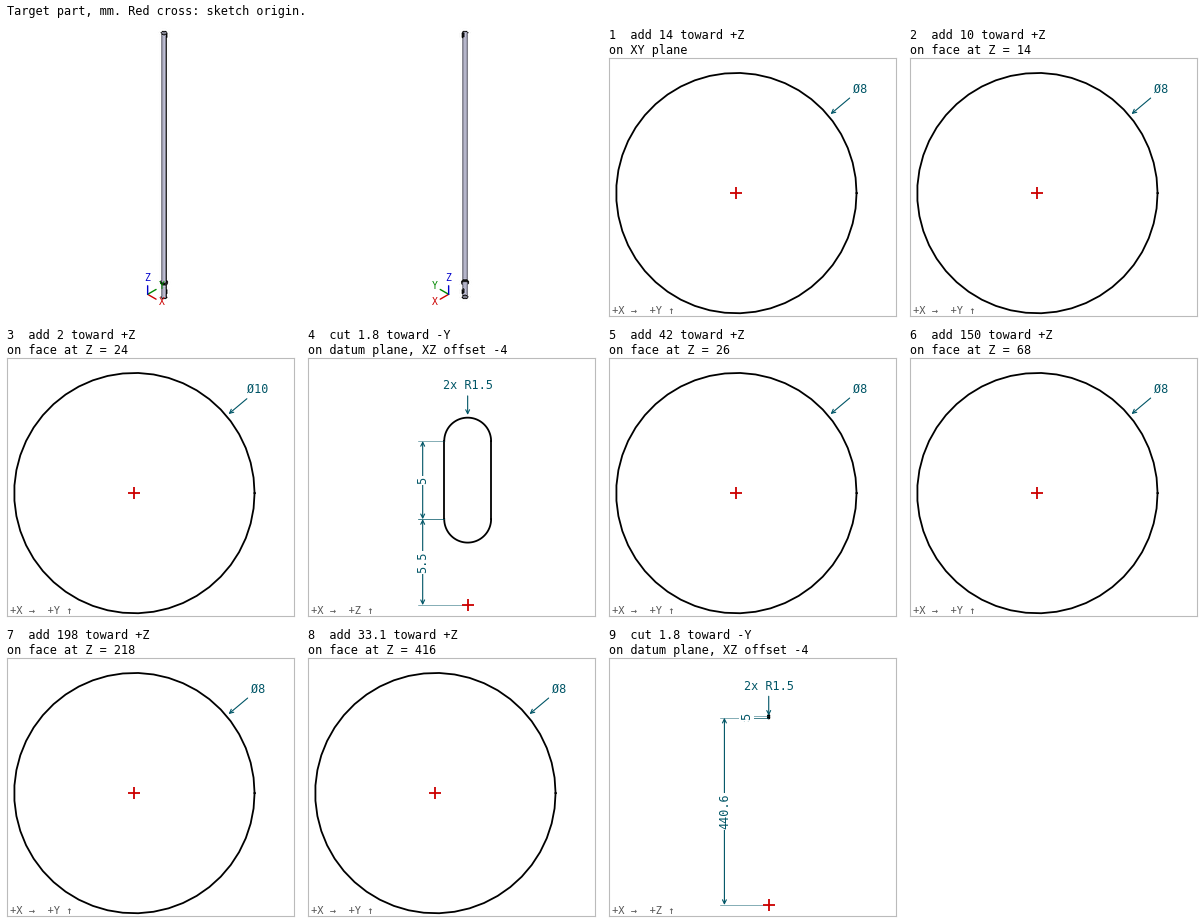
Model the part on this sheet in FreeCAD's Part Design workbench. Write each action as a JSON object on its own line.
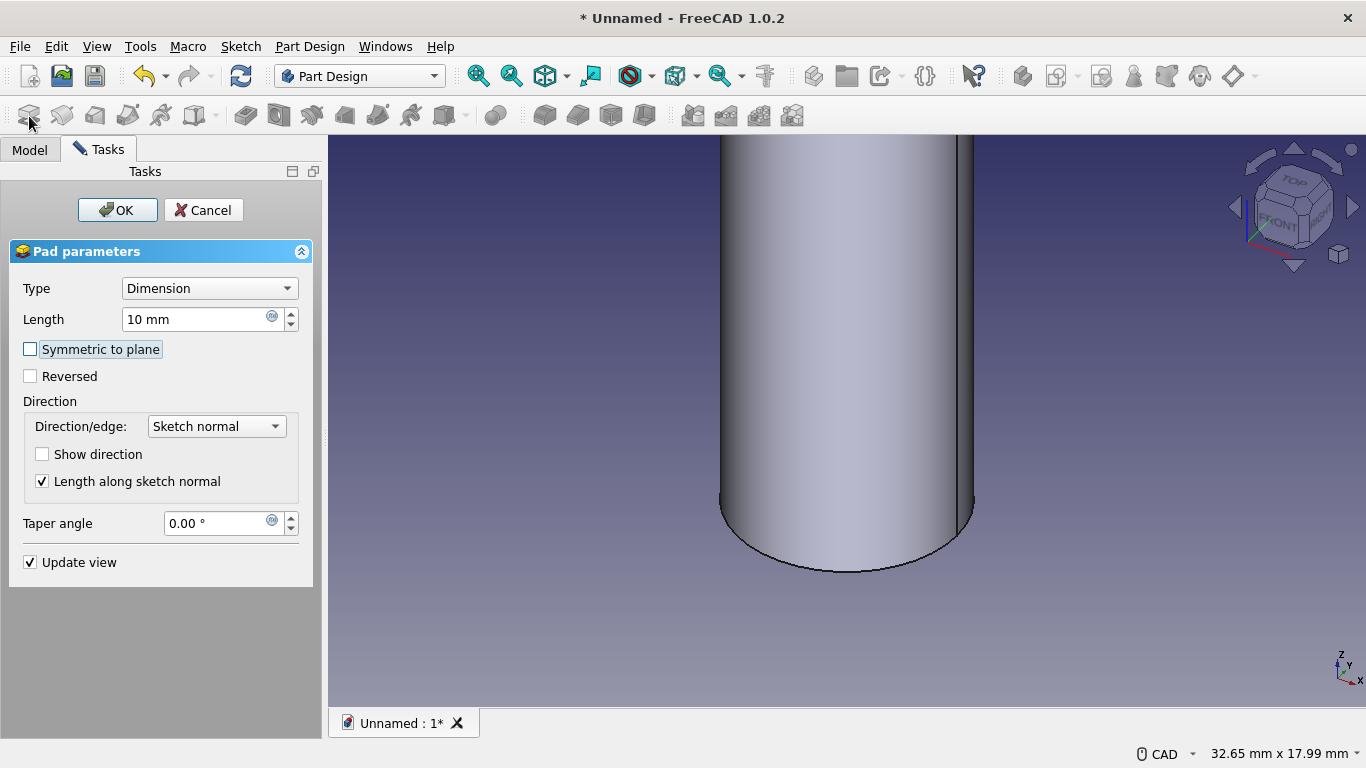
{"action": "left_click", "coordinate": [118, 210]}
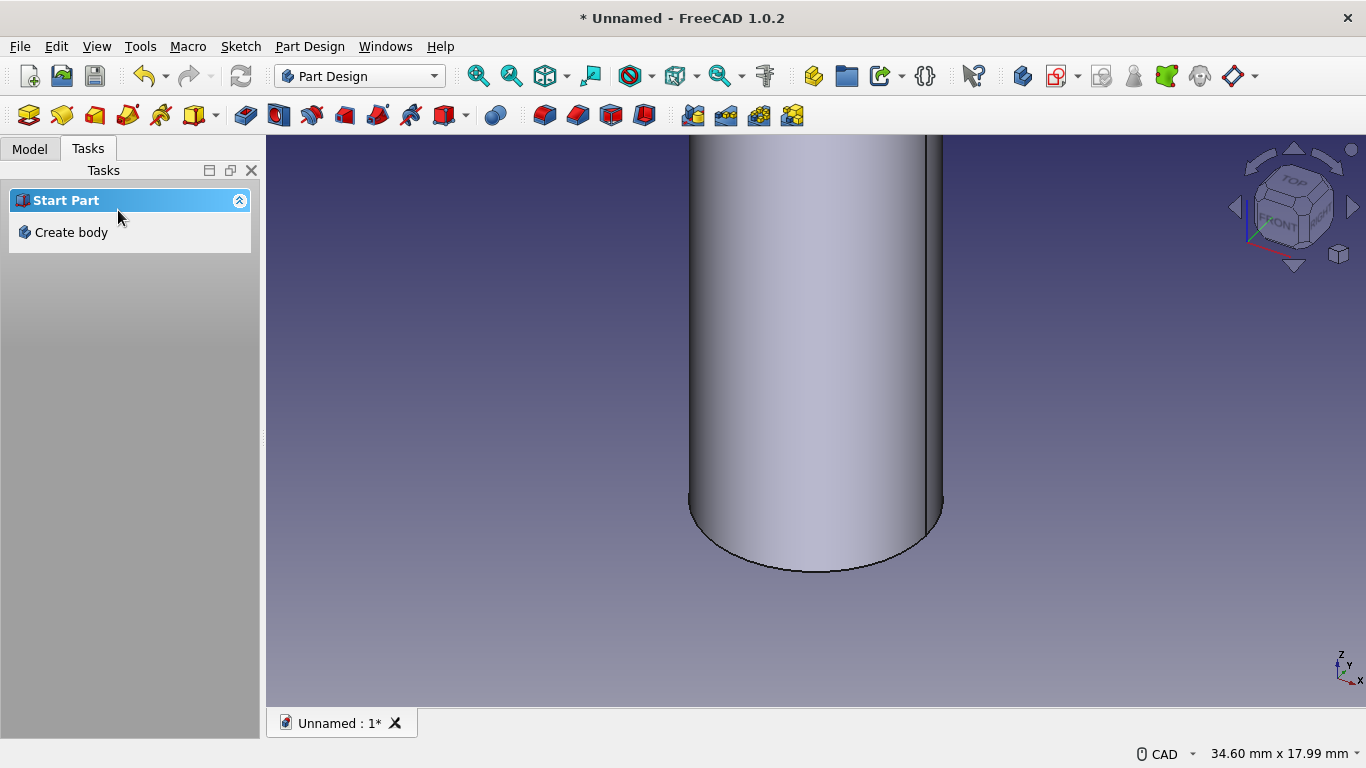
{"action": "left_click", "coordinate": [479, 76]}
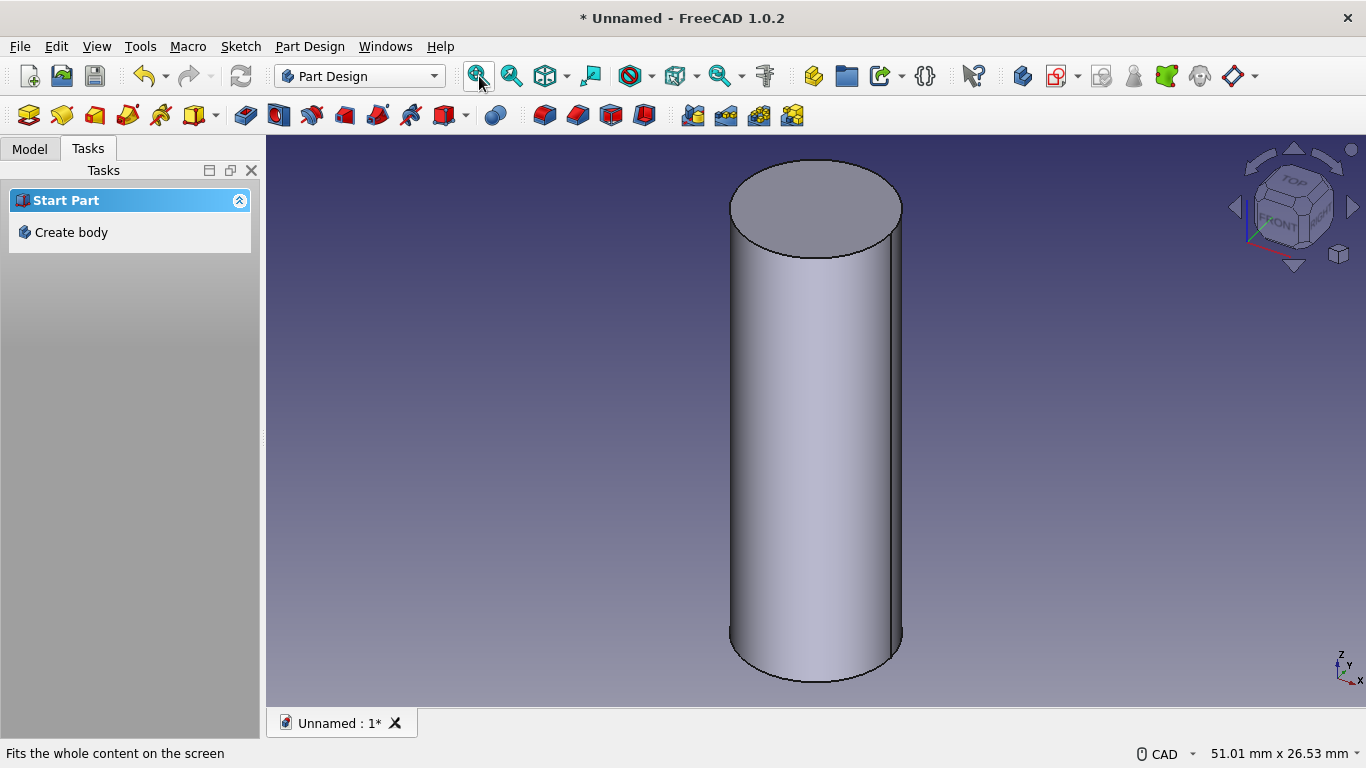
{"action": "left_click", "coordinate": [816, 208]}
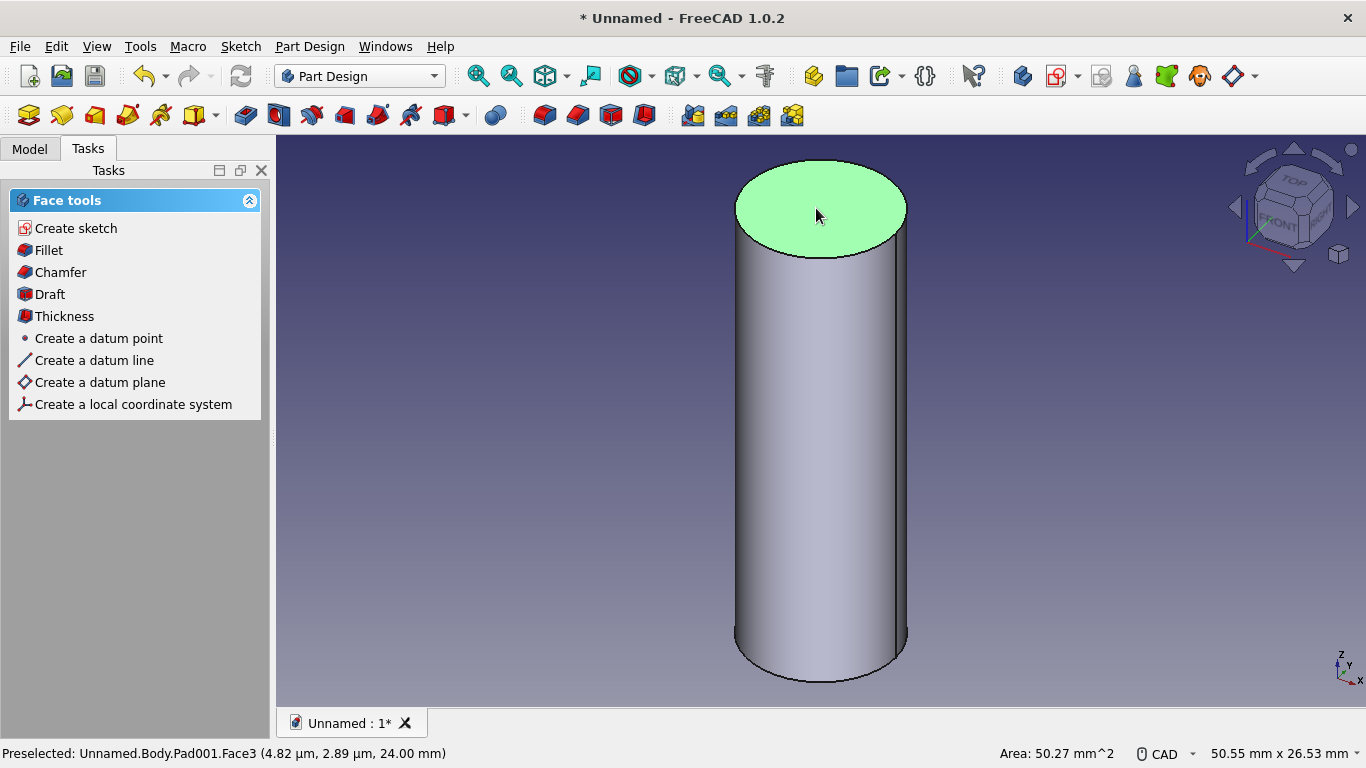
{"action": "left_click", "coordinate": [1056, 76]}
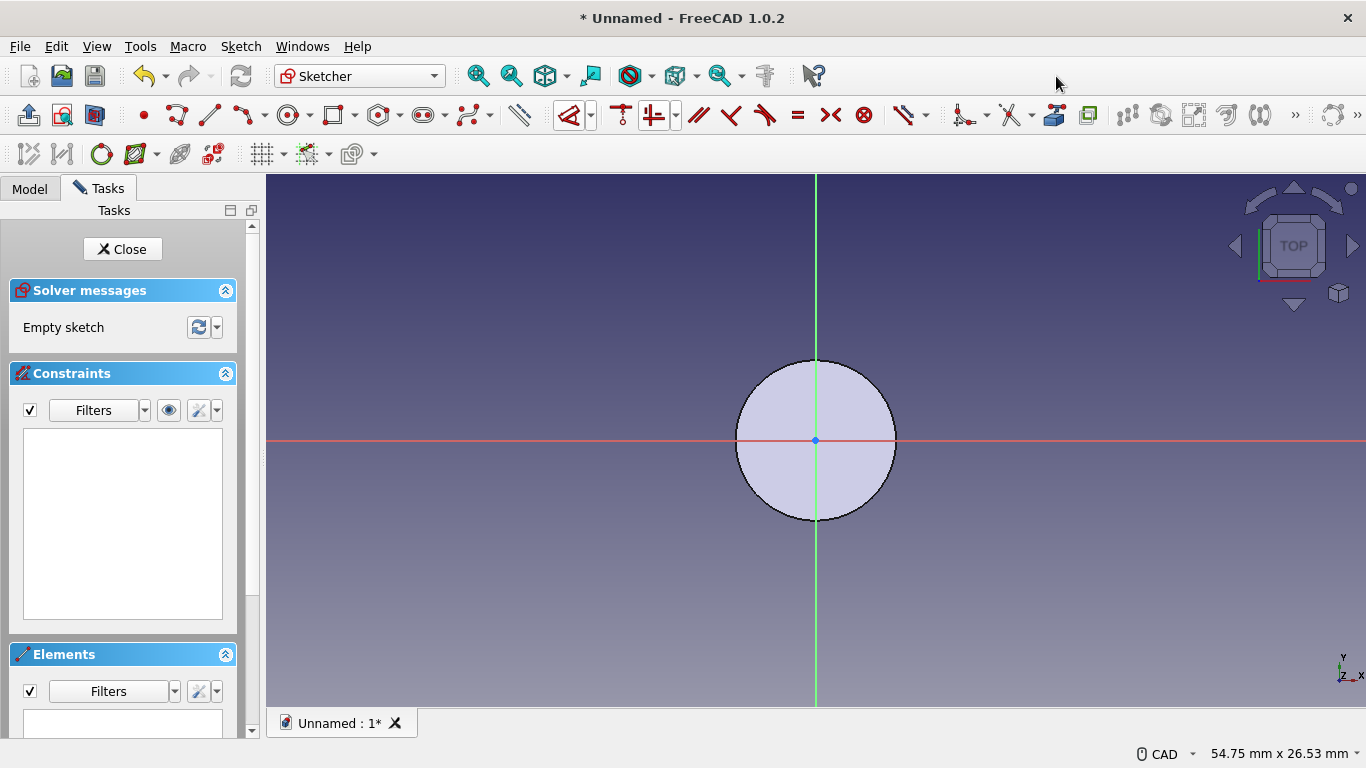
{"action": "scroll", "coordinate": [899, 441], "scroll_direction": "up", "scroll_amount": 3}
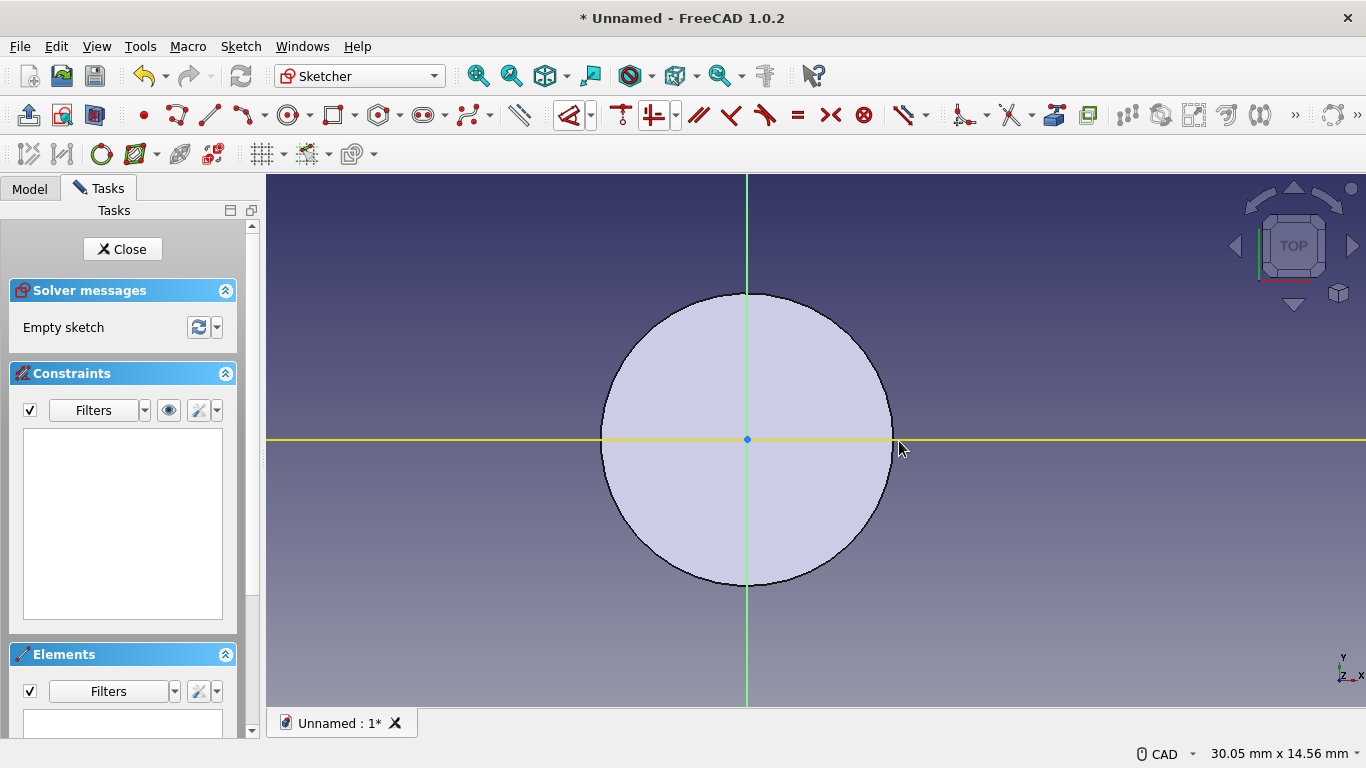
{"action": "left_click", "coordinate": [288, 116]}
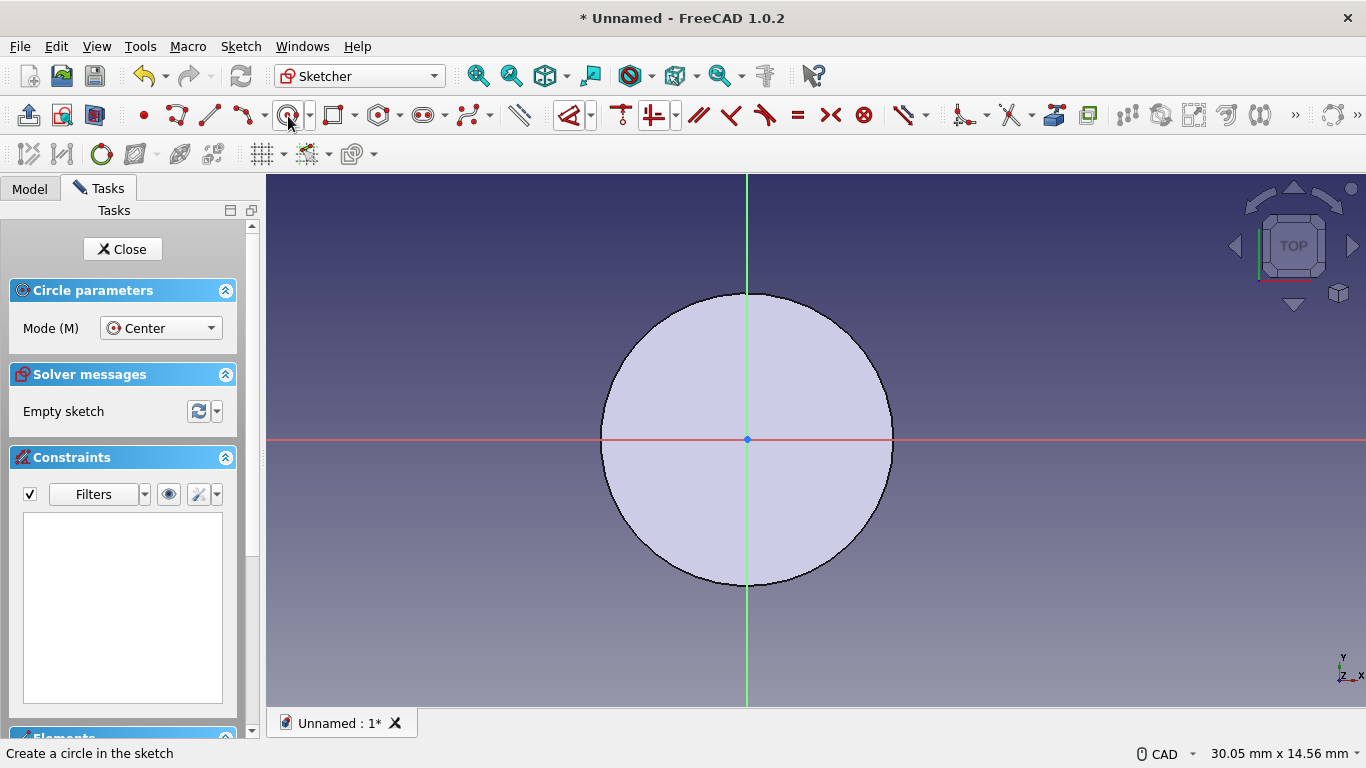
{"action": "left_click", "coordinate": [747, 440]}
{"action": "left_click", "coordinate": [876, 310]}
{"action": "key", "text": "Escape"}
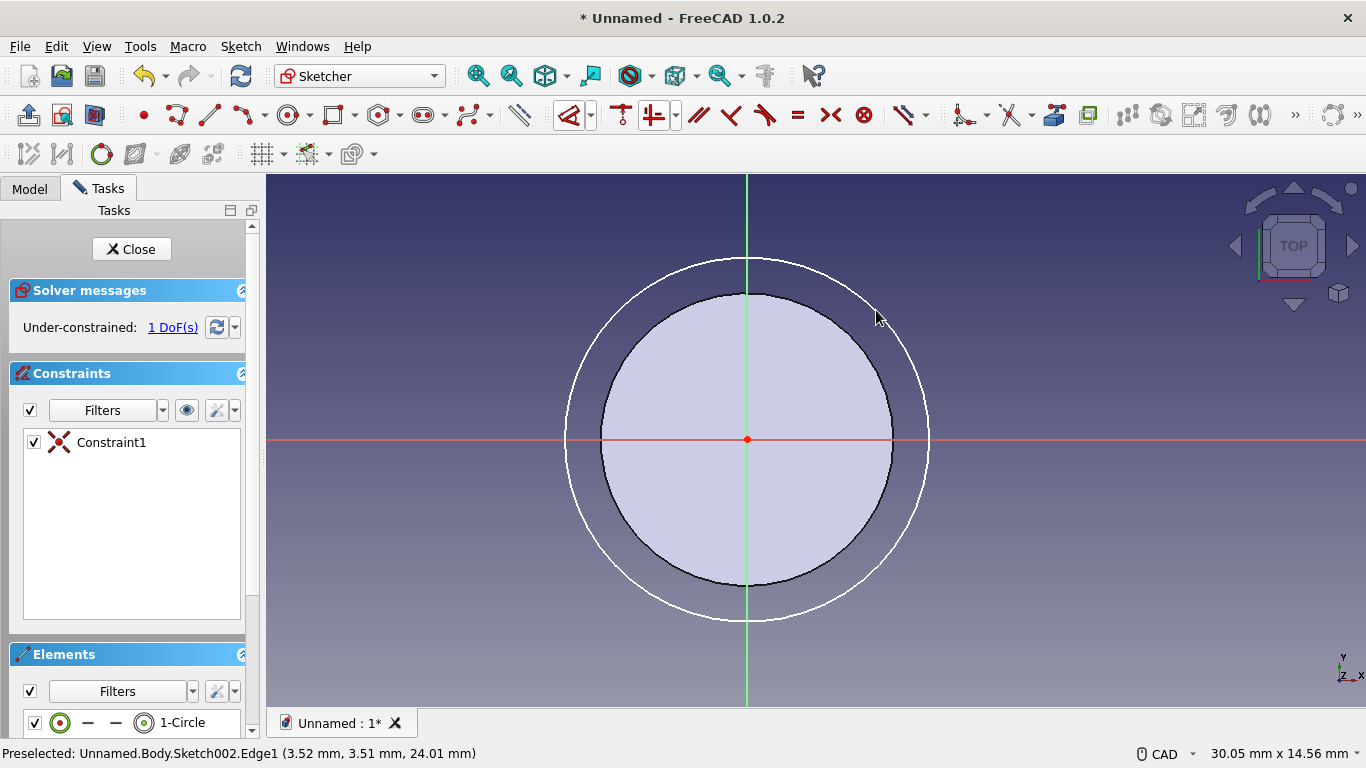
{"action": "left_click", "coordinate": [875, 310]}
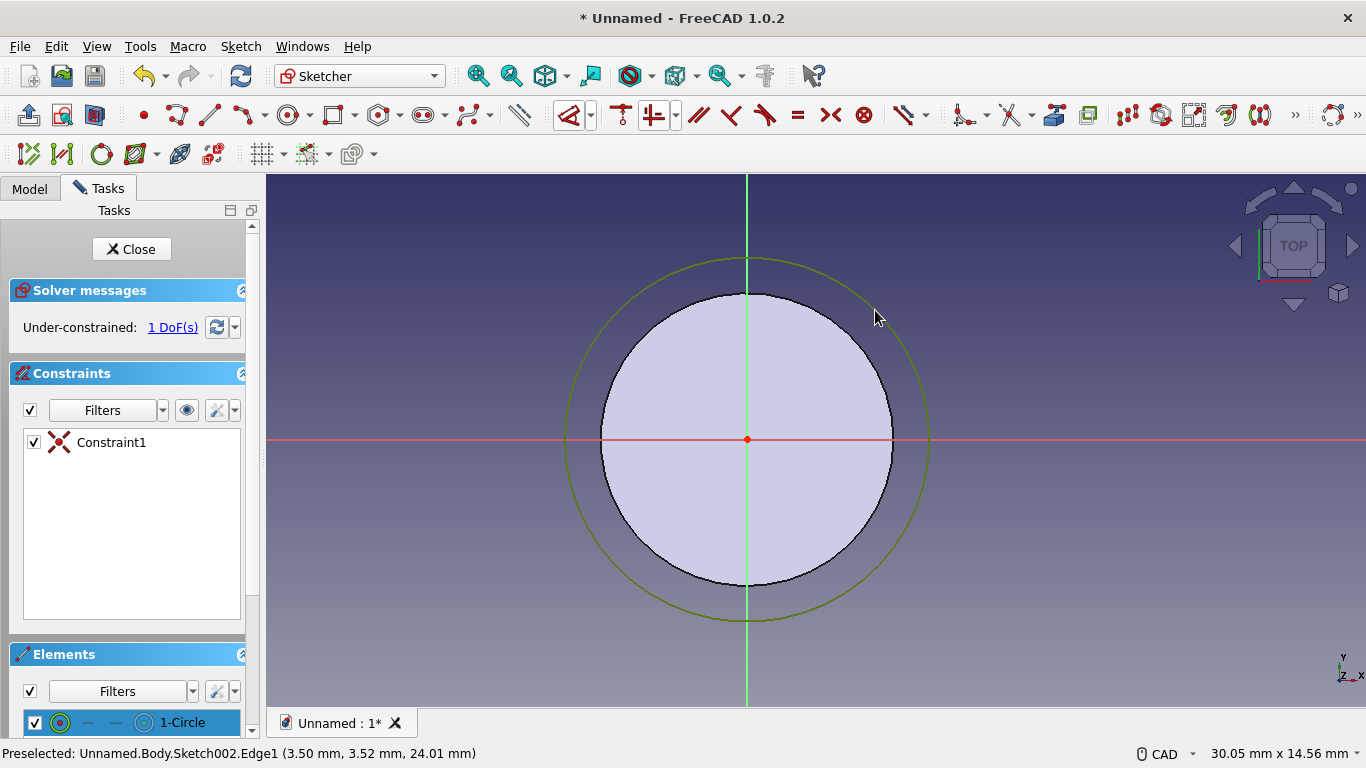
{"action": "left_click", "coordinate": [590, 116]}